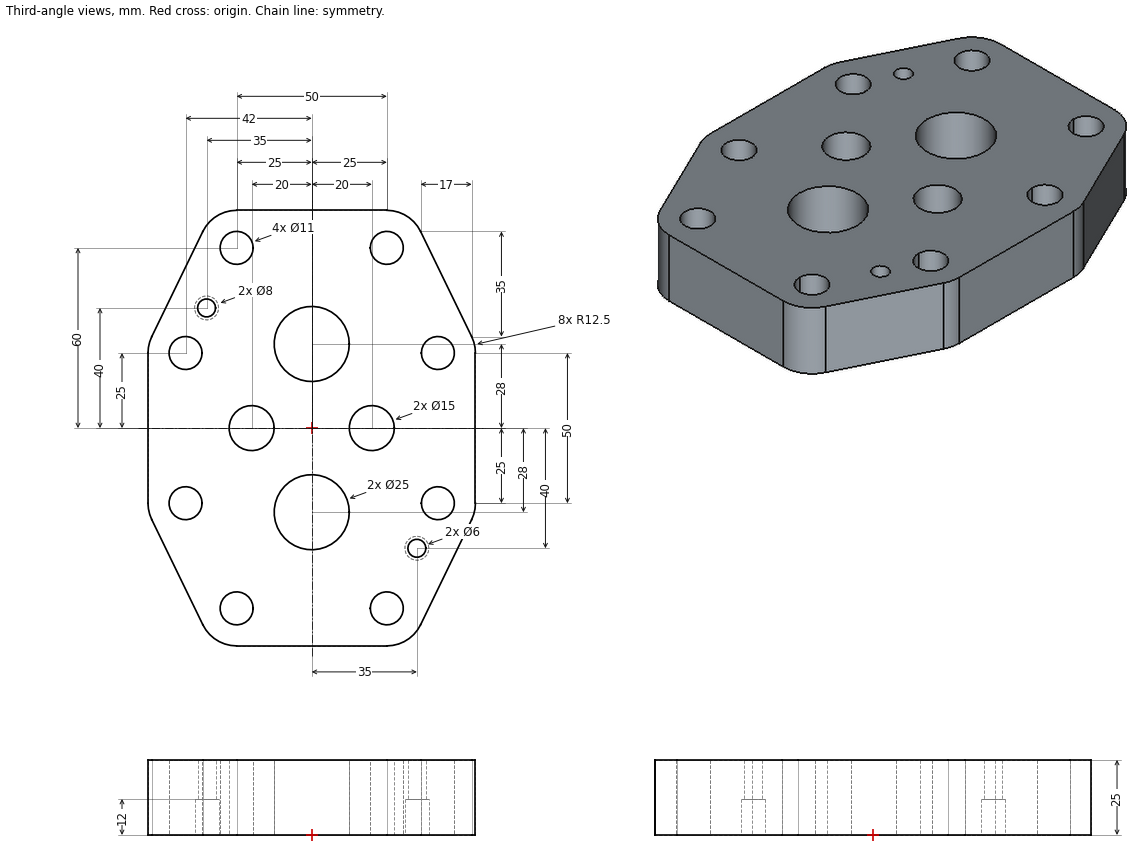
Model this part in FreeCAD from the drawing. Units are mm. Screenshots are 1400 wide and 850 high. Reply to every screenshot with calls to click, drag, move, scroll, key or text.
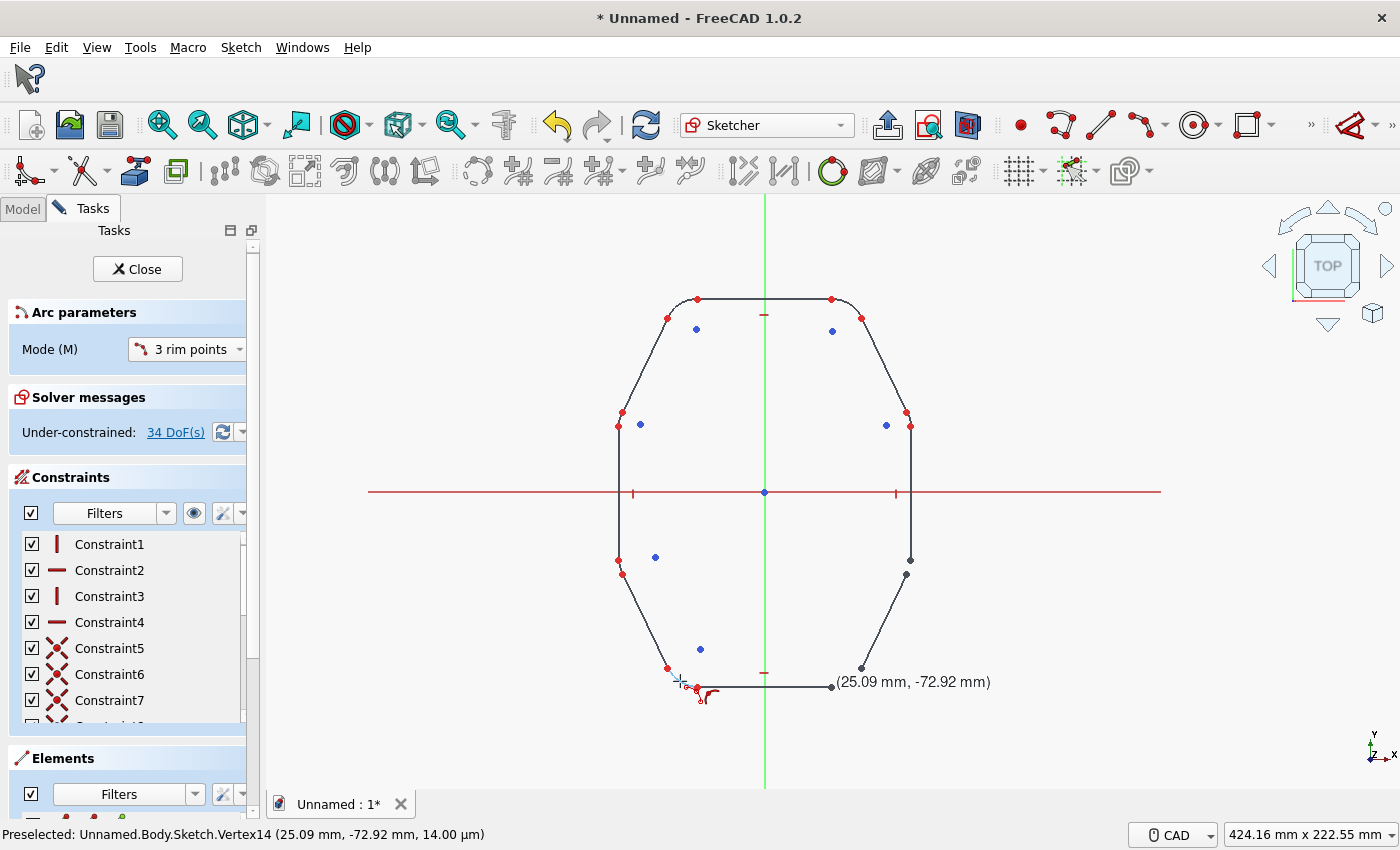
click(862, 668)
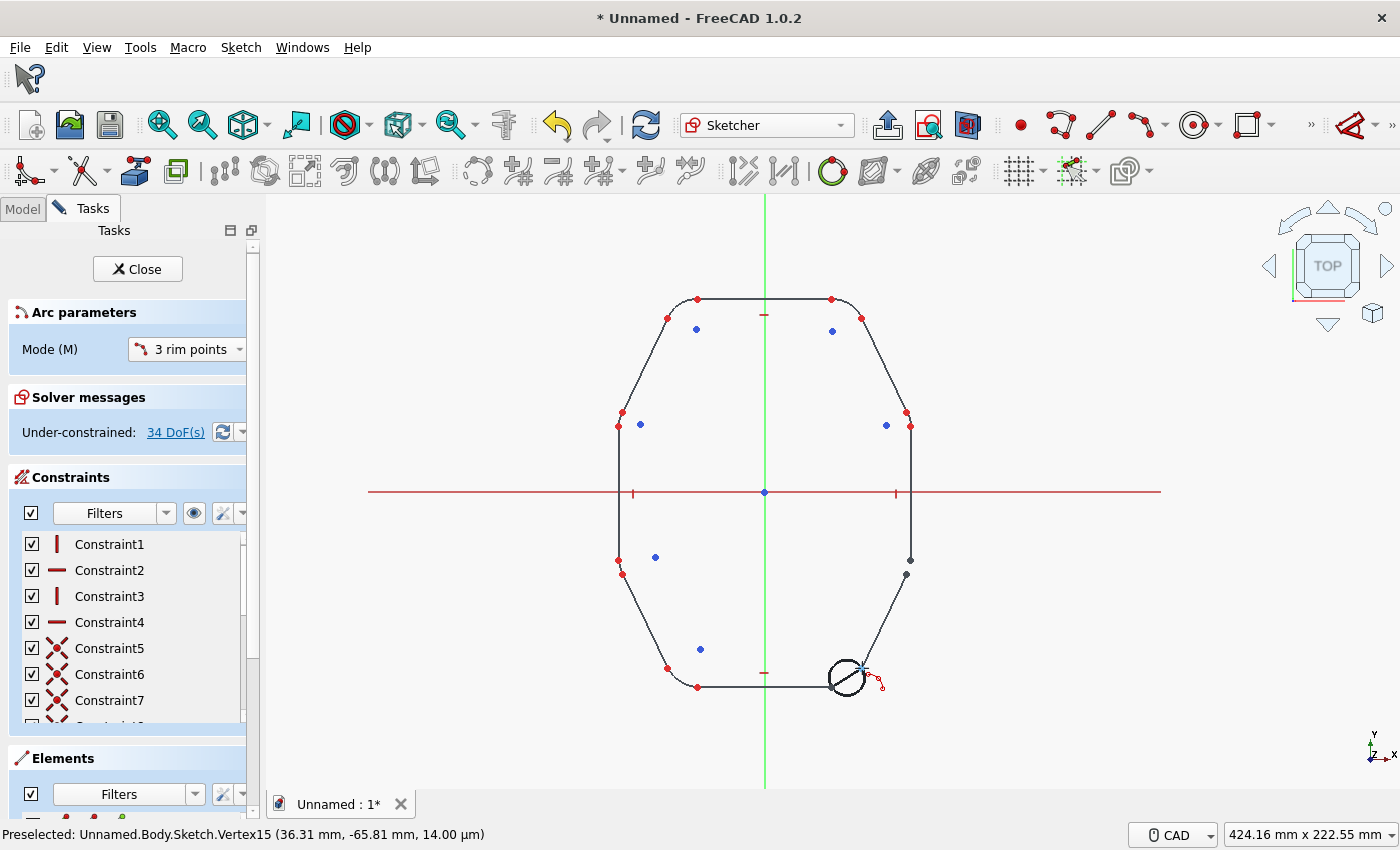
scroll(849, 681, up, 6)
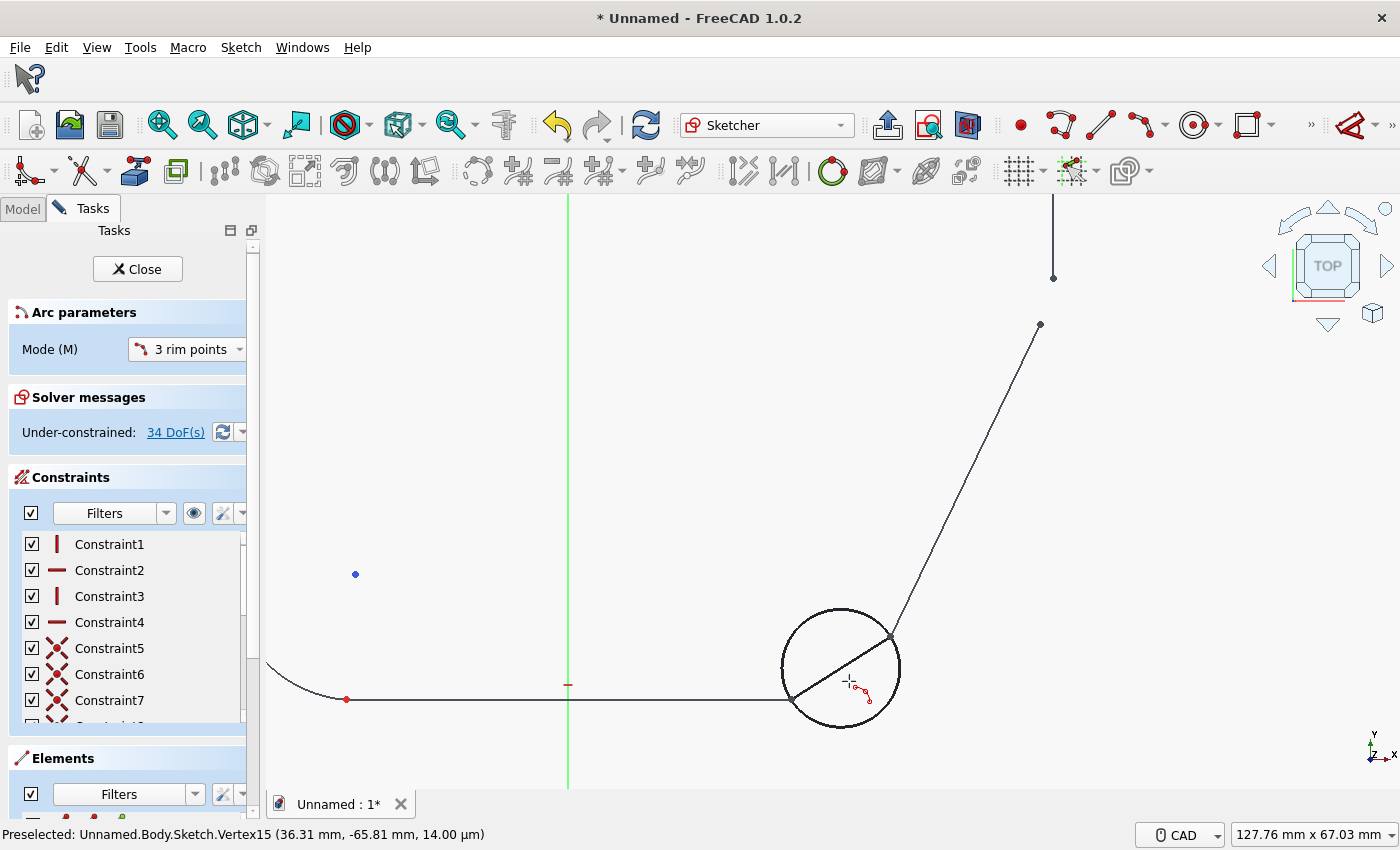
click(849, 679)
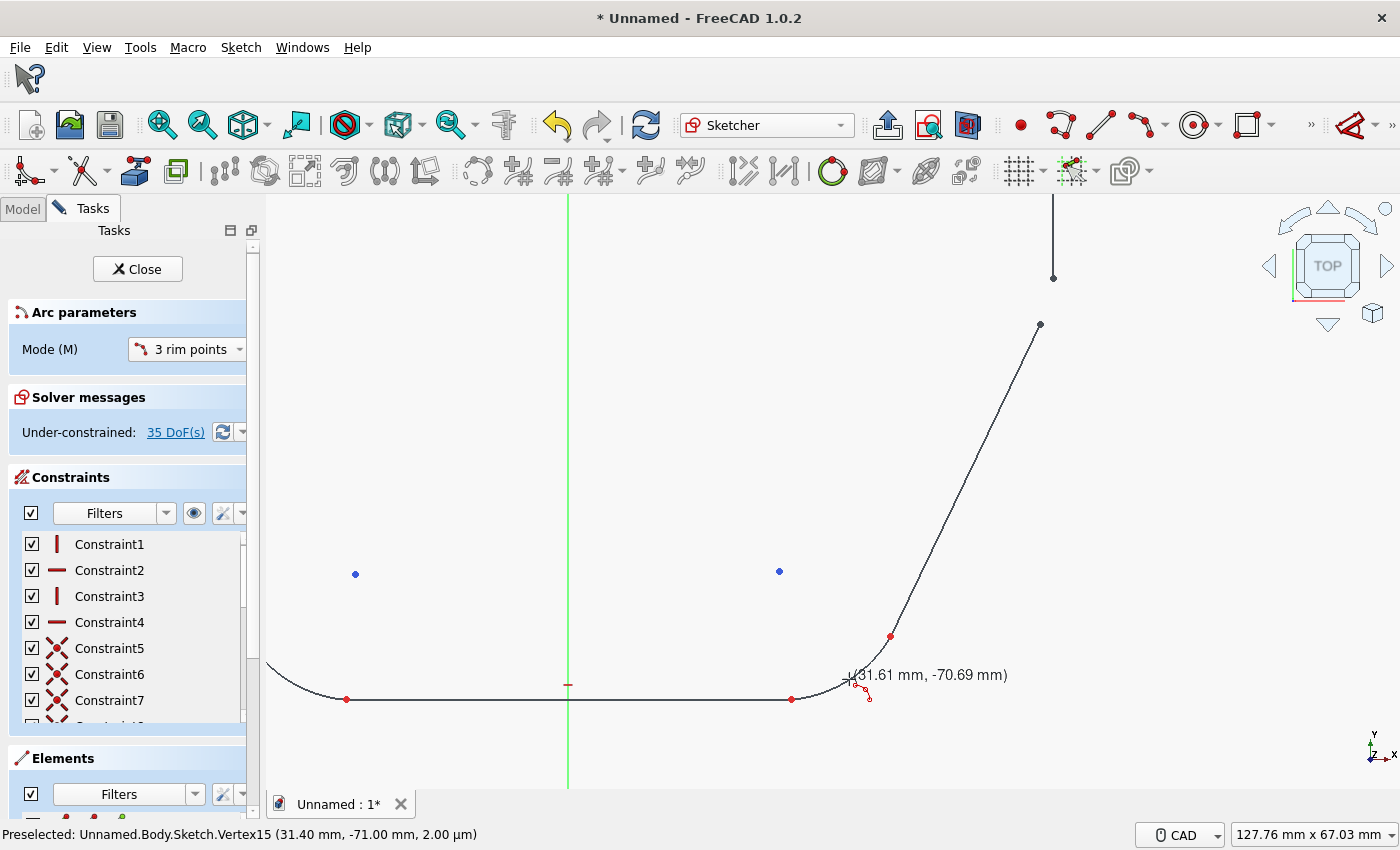
click(1040, 325)
click(1053, 278)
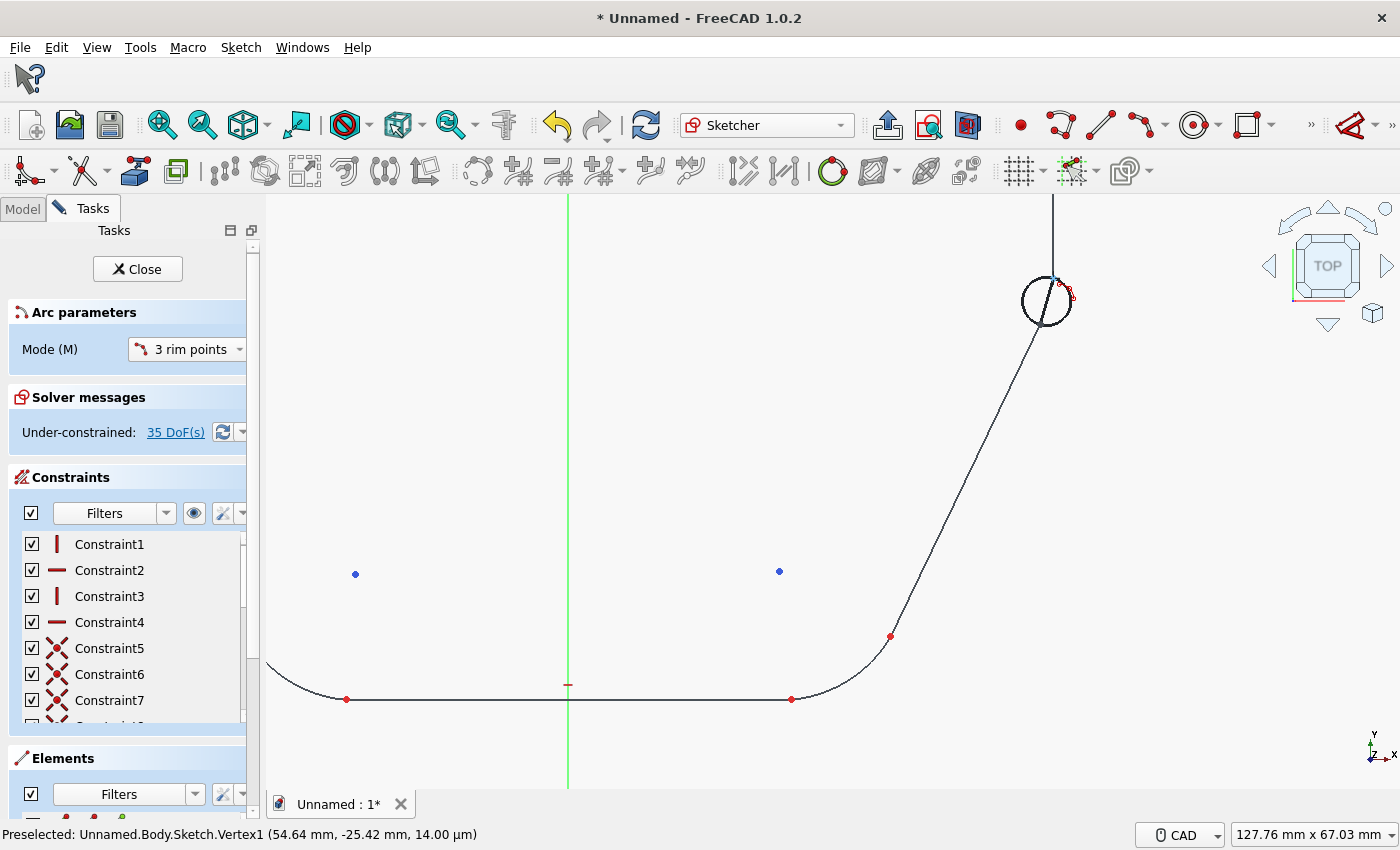
scroll(1049, 299, up, 9)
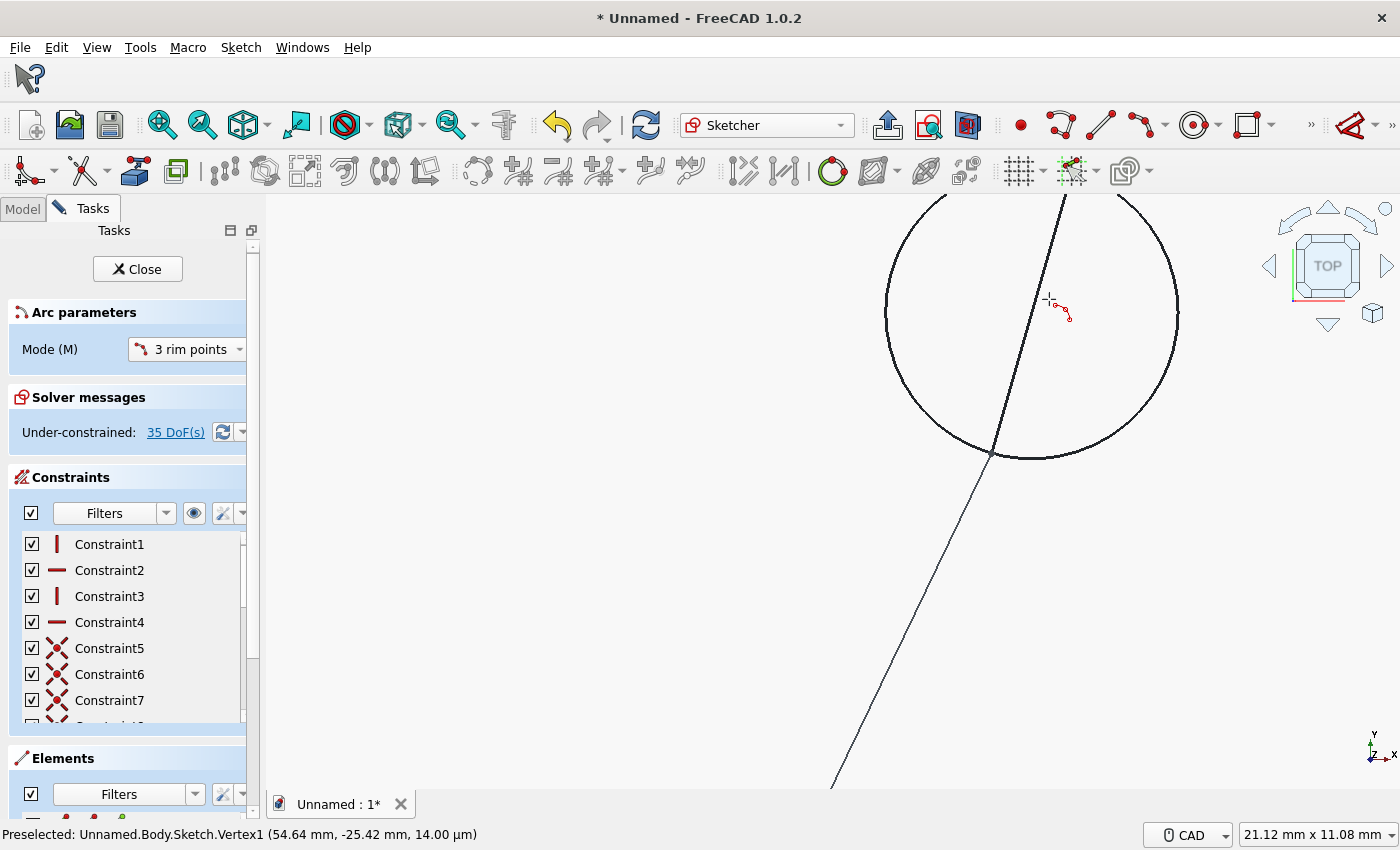
click(1048, 300)
key(Escape)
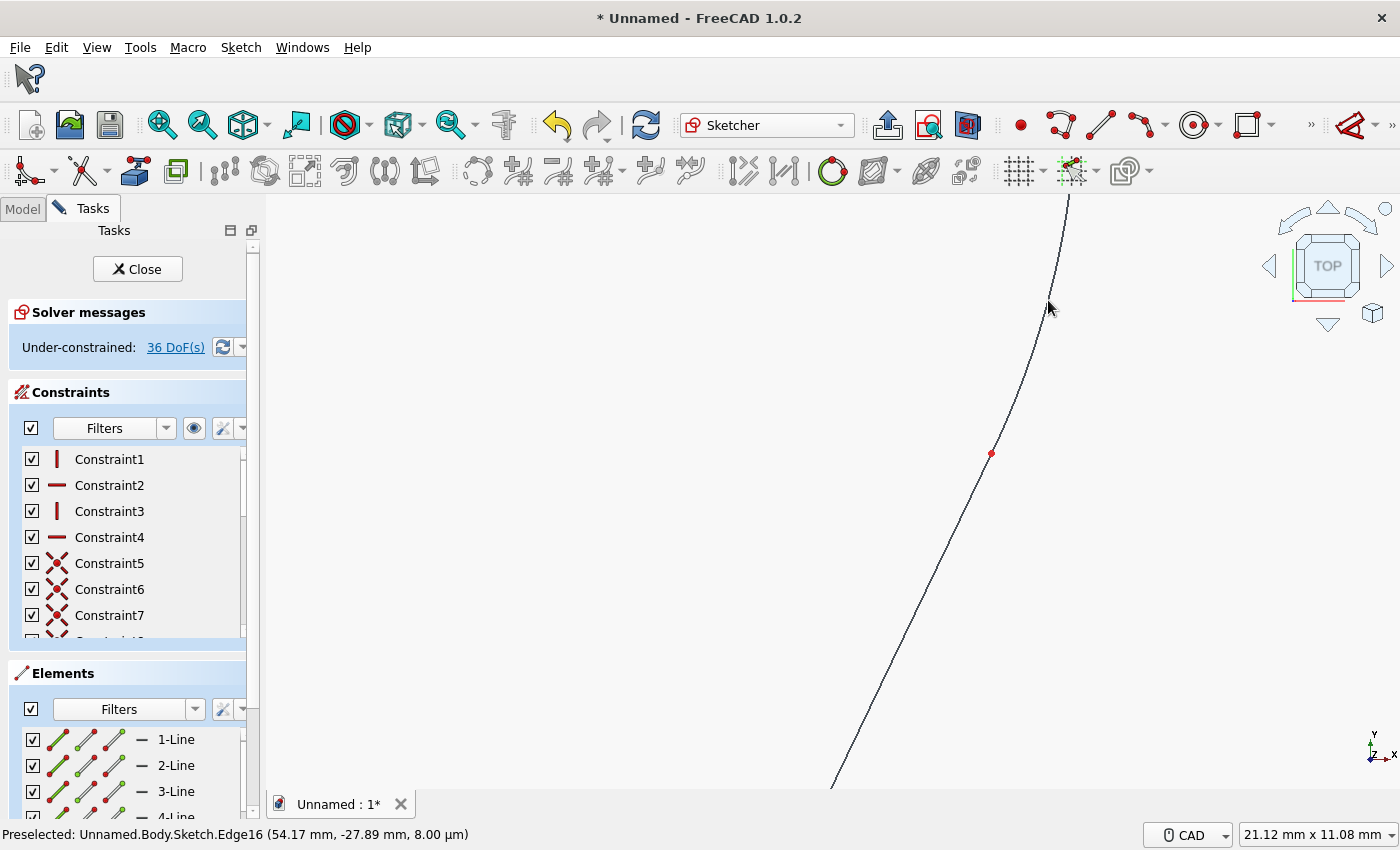
scroll(902, 580, down, 15)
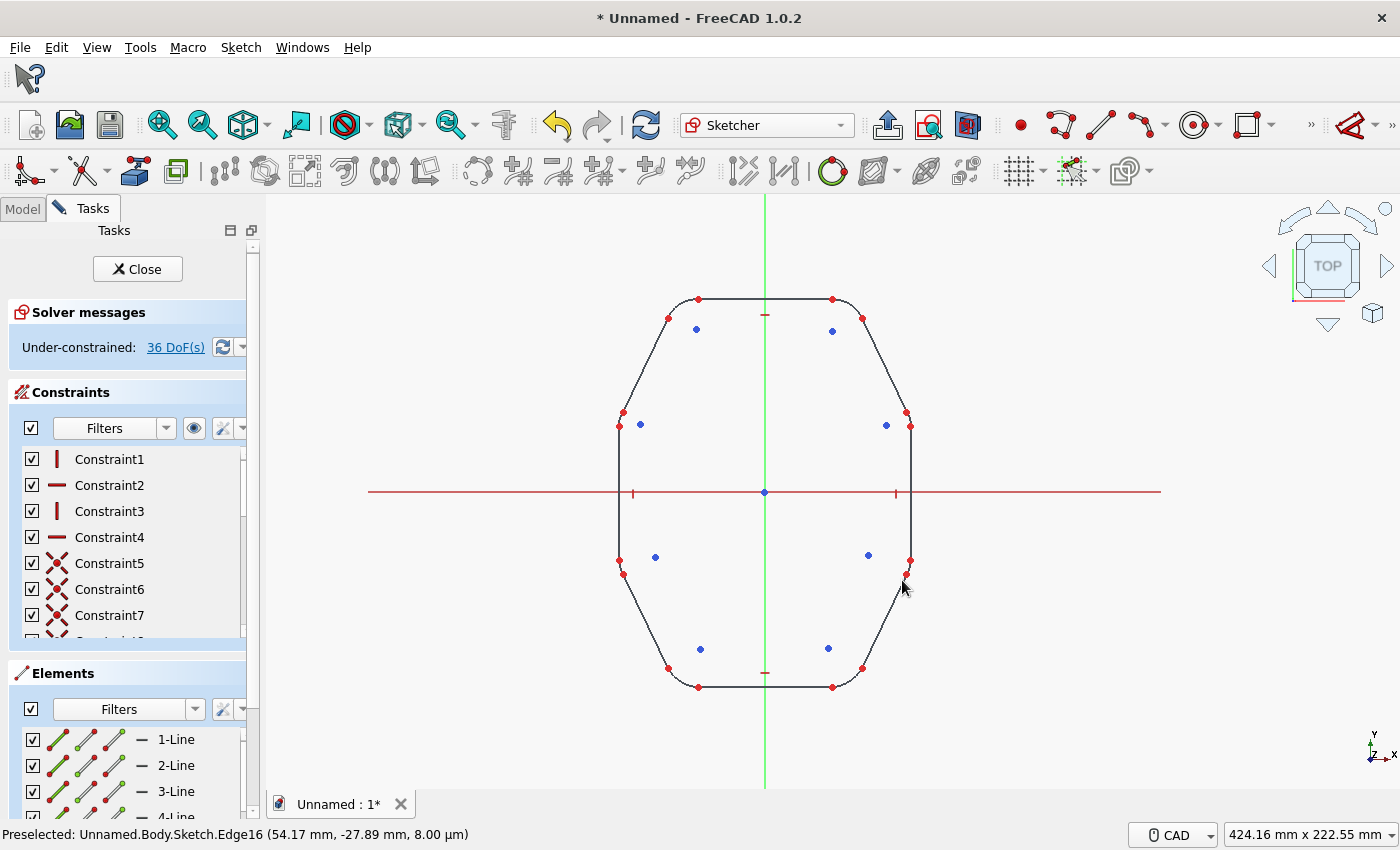
click(911, 520)